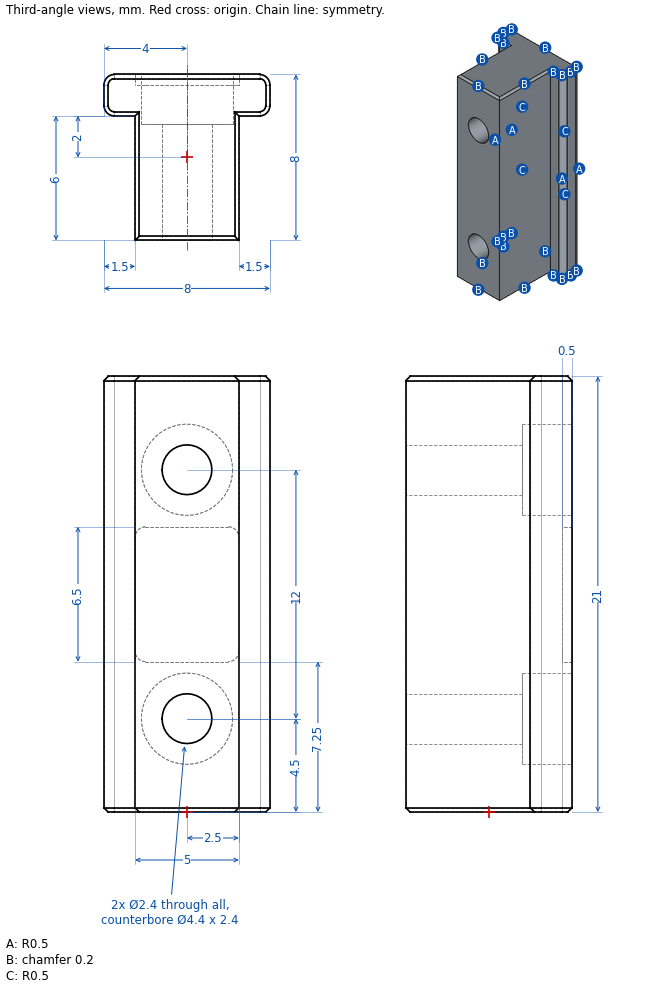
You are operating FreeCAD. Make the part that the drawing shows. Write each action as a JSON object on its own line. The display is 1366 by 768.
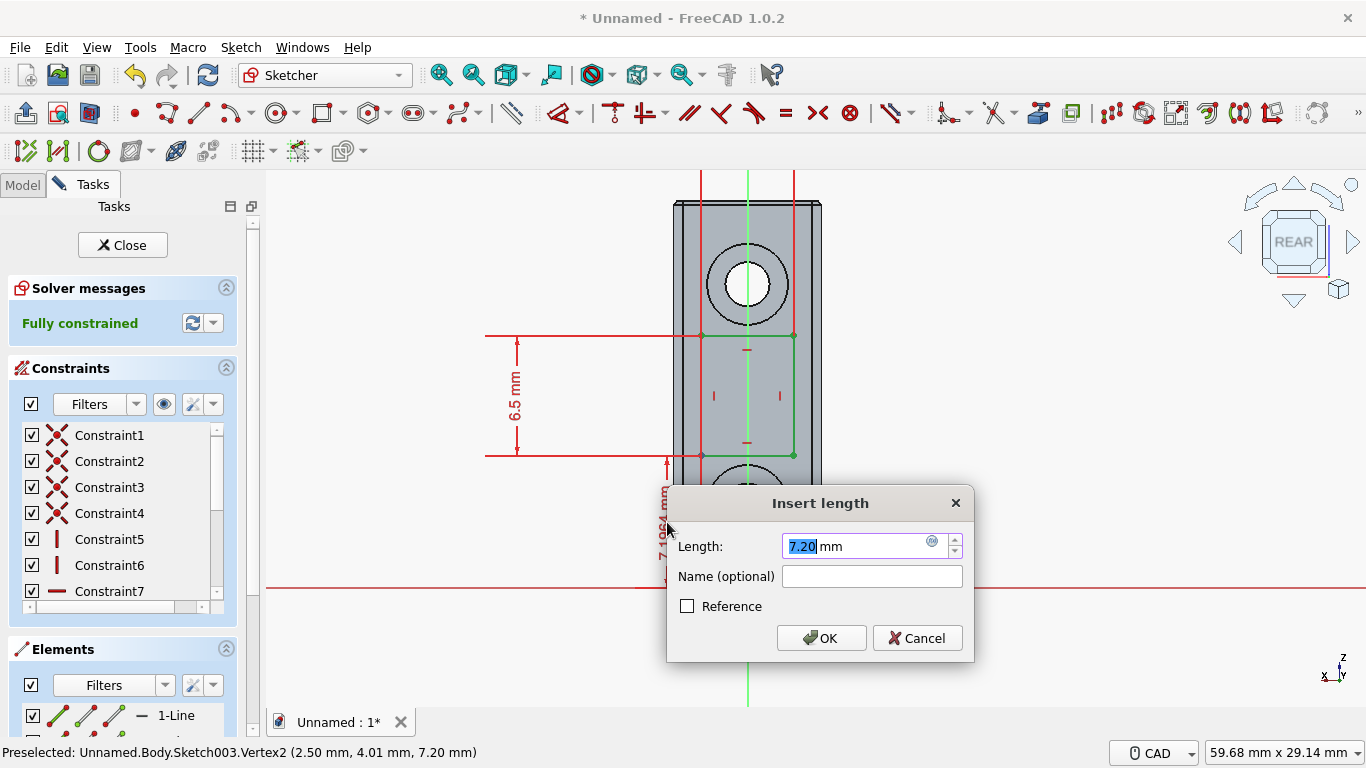
{"action": "type", "text": "7.25"}
{"action": "key", "text": "Return"}
{"action": "key", "text": "Escape"}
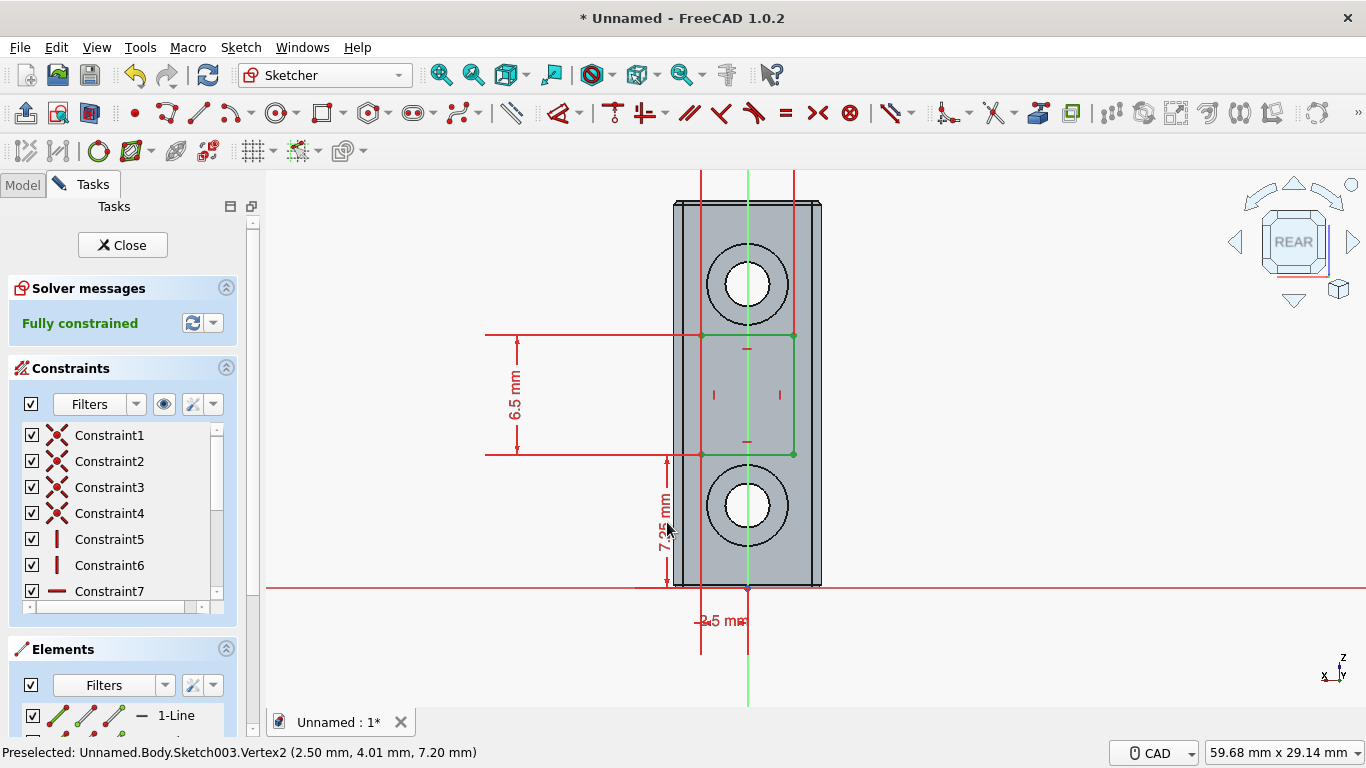
{"action": "left_click", "coordinate": [123, 245]}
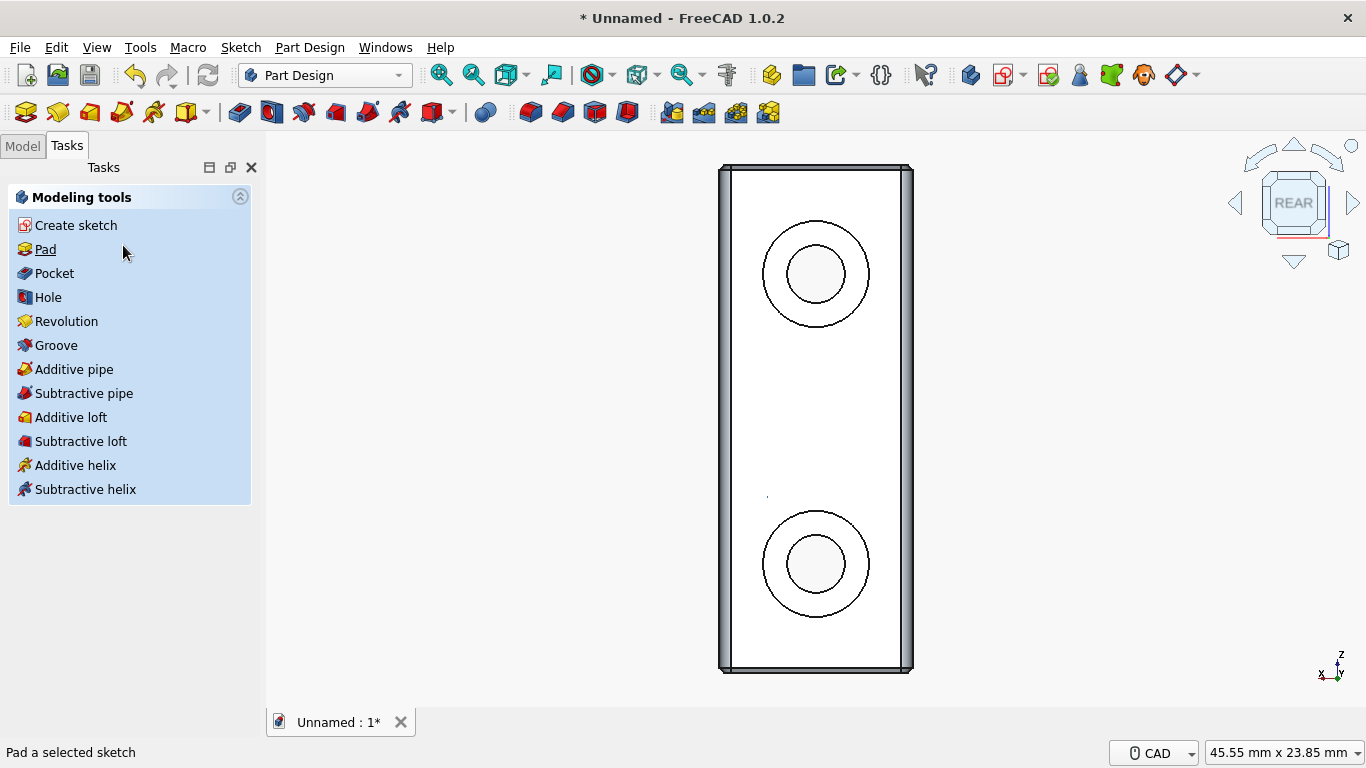
{"action": "left_click", "coordinate": [240, 112]}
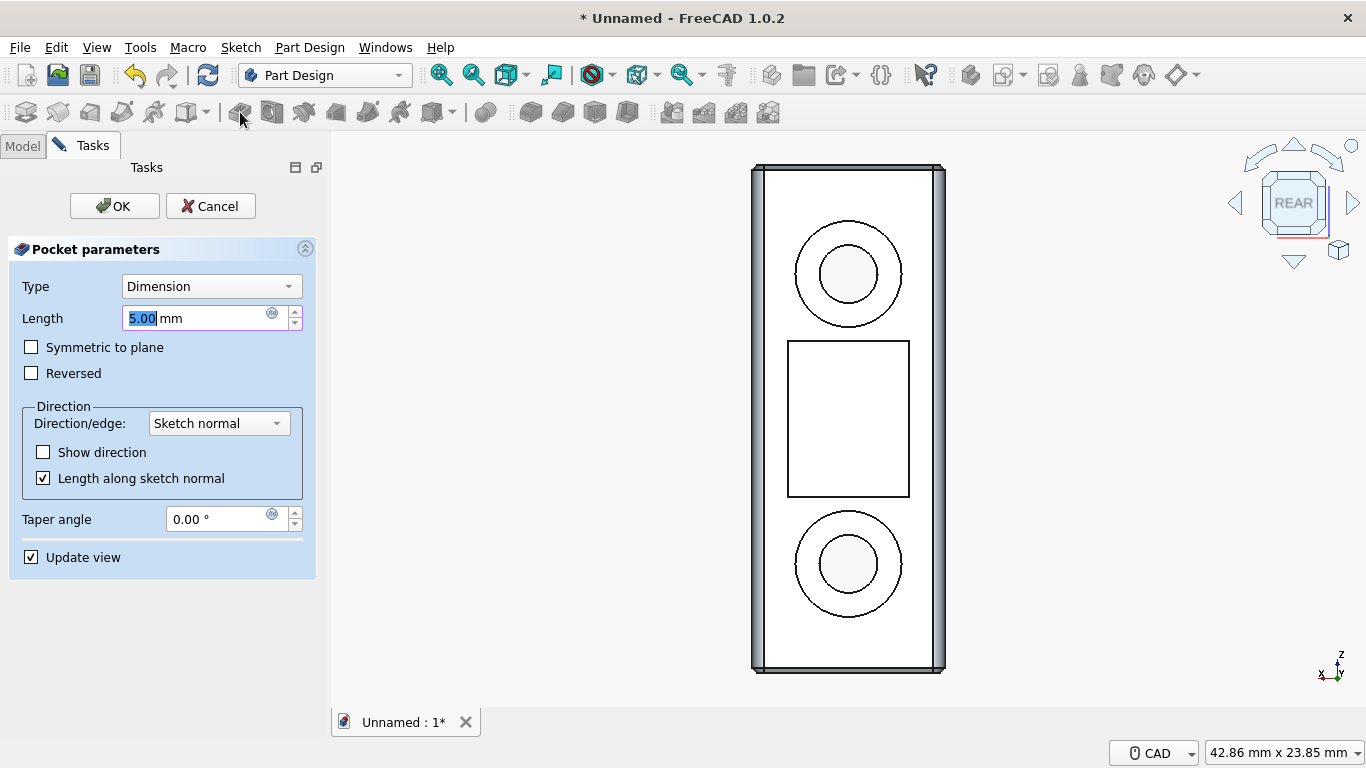
{"action": "type", "text": "0.5"}
{"action": "key", "text": "Tab"}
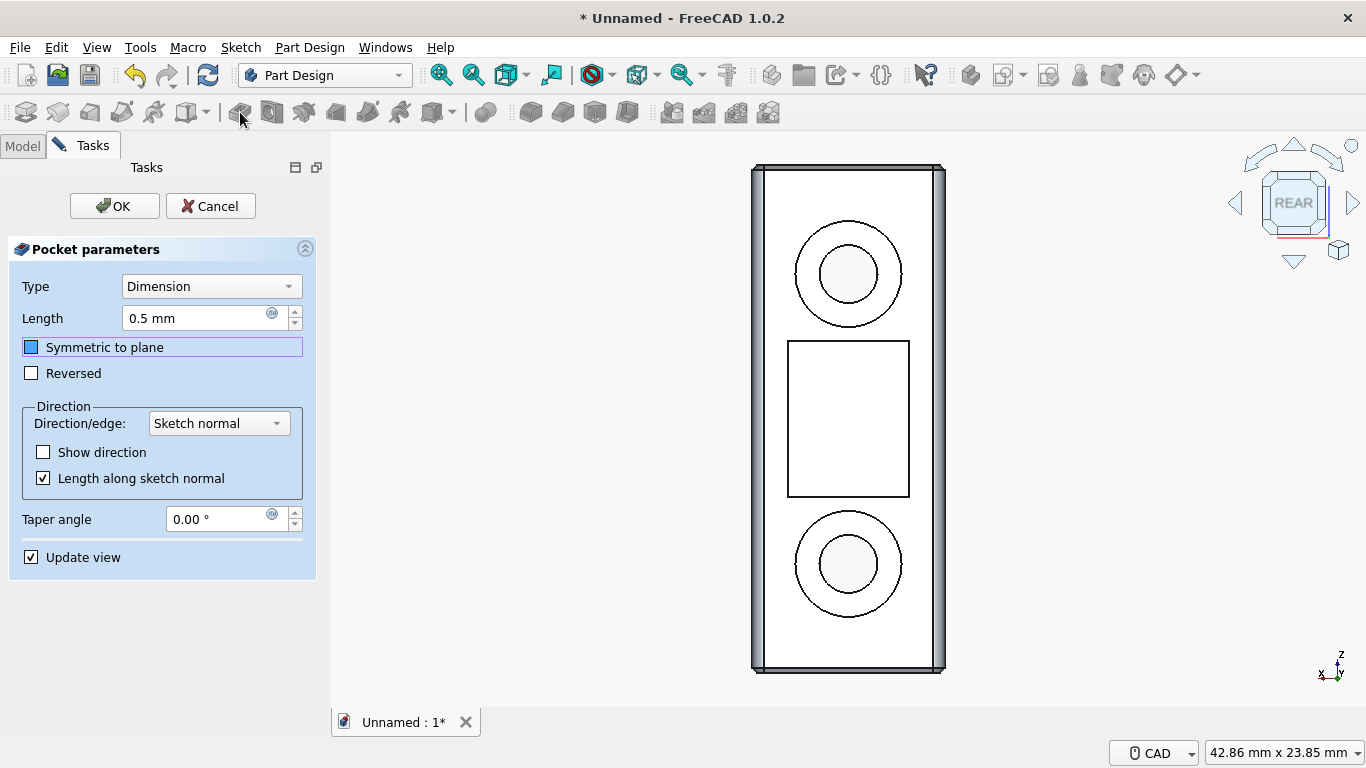
{"action": "left_click", "coordinate": [115, 206]}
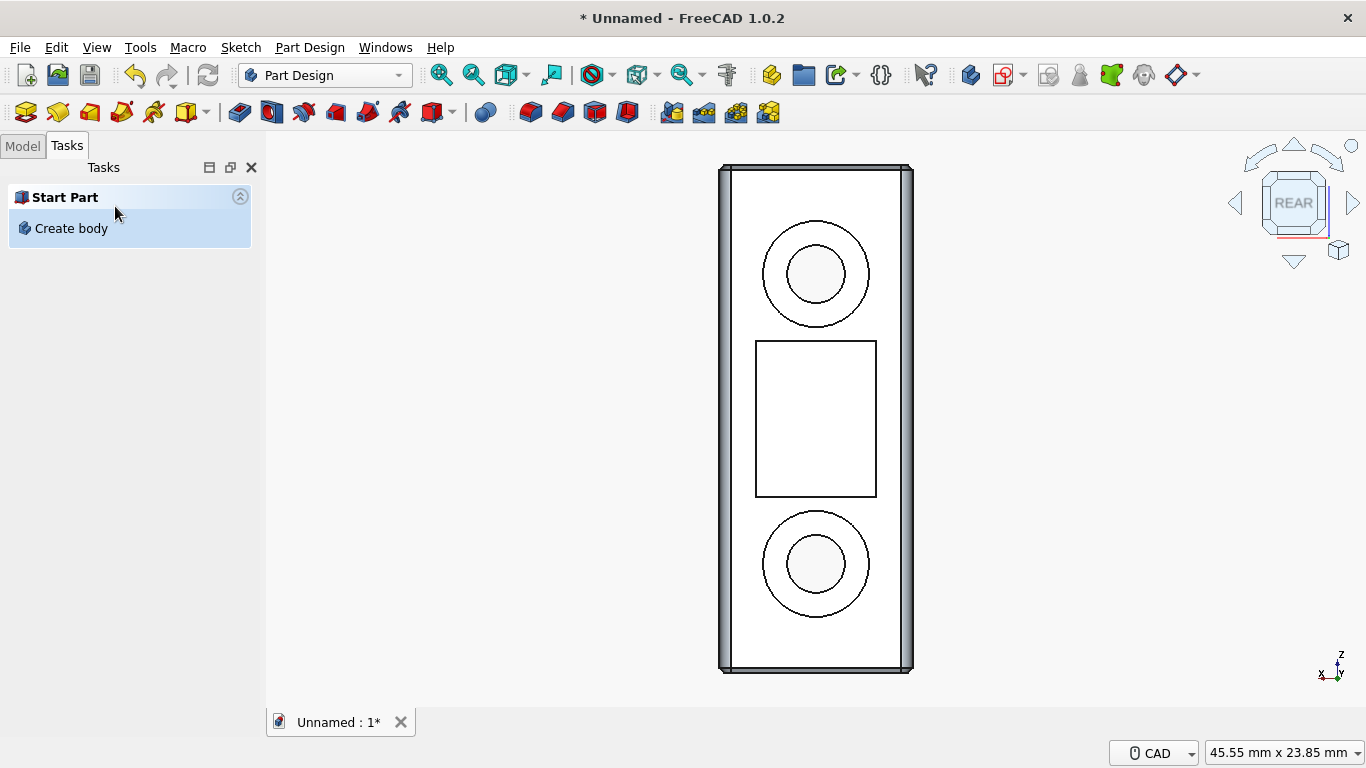
{"action": "scroll", "coordinate": [756, 496], "scroll_direction": "up", "scroll_amount": 6}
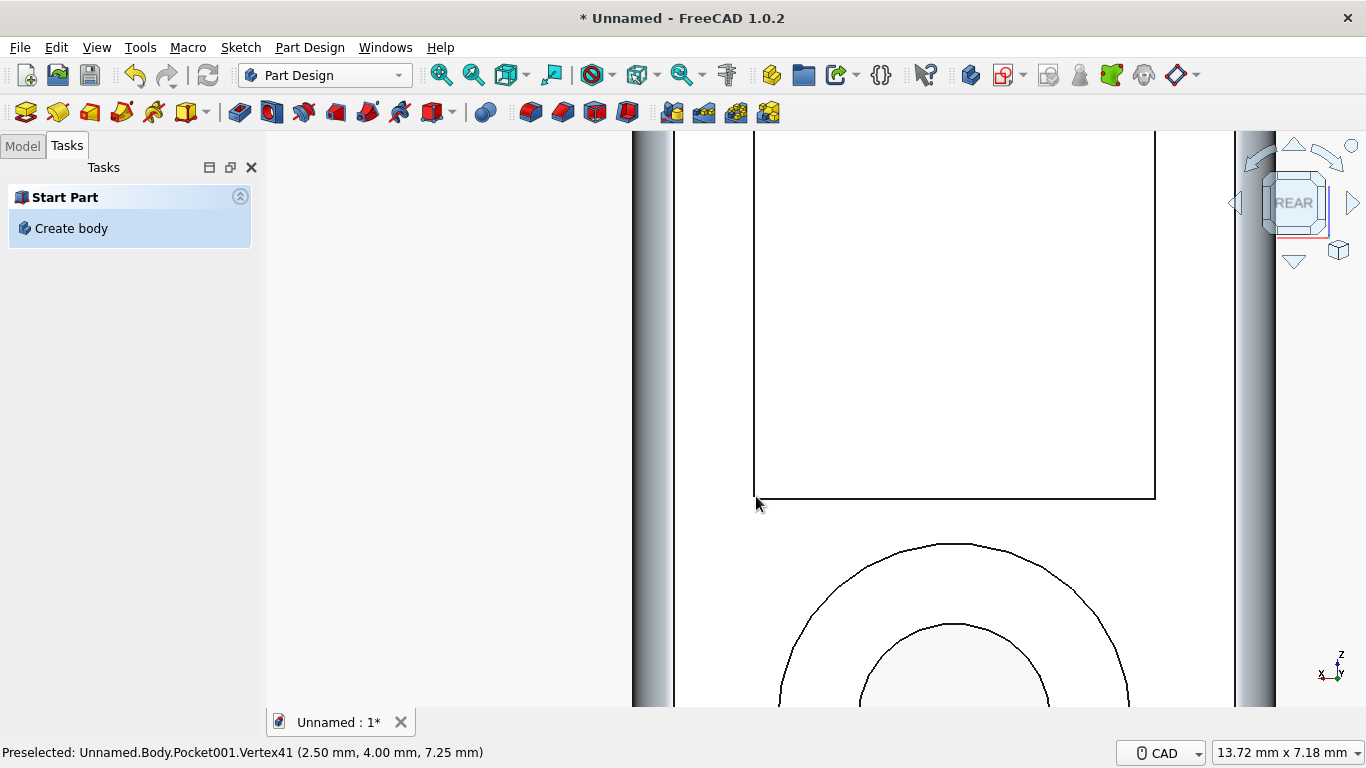
{"action": "left_click", "coordinate": [442, 76]}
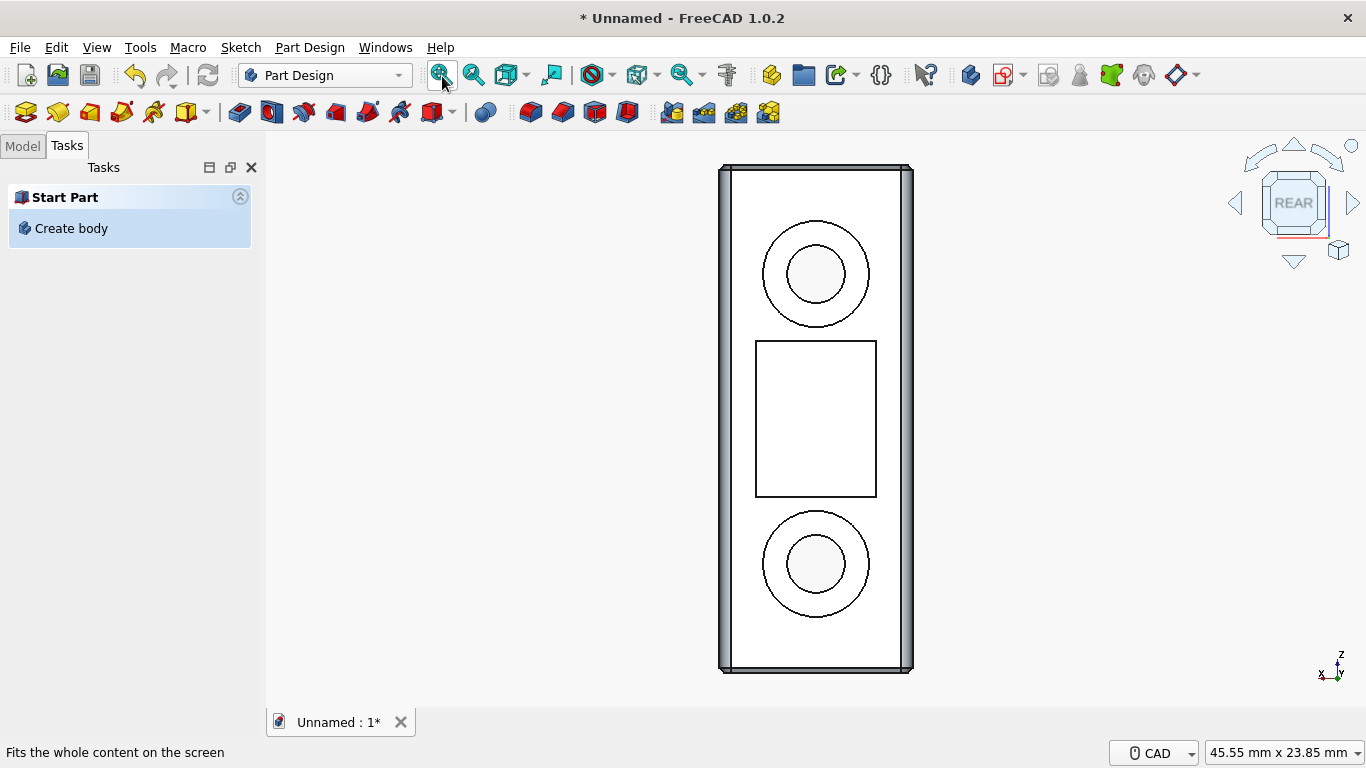
{"action": "key", "text": "0"}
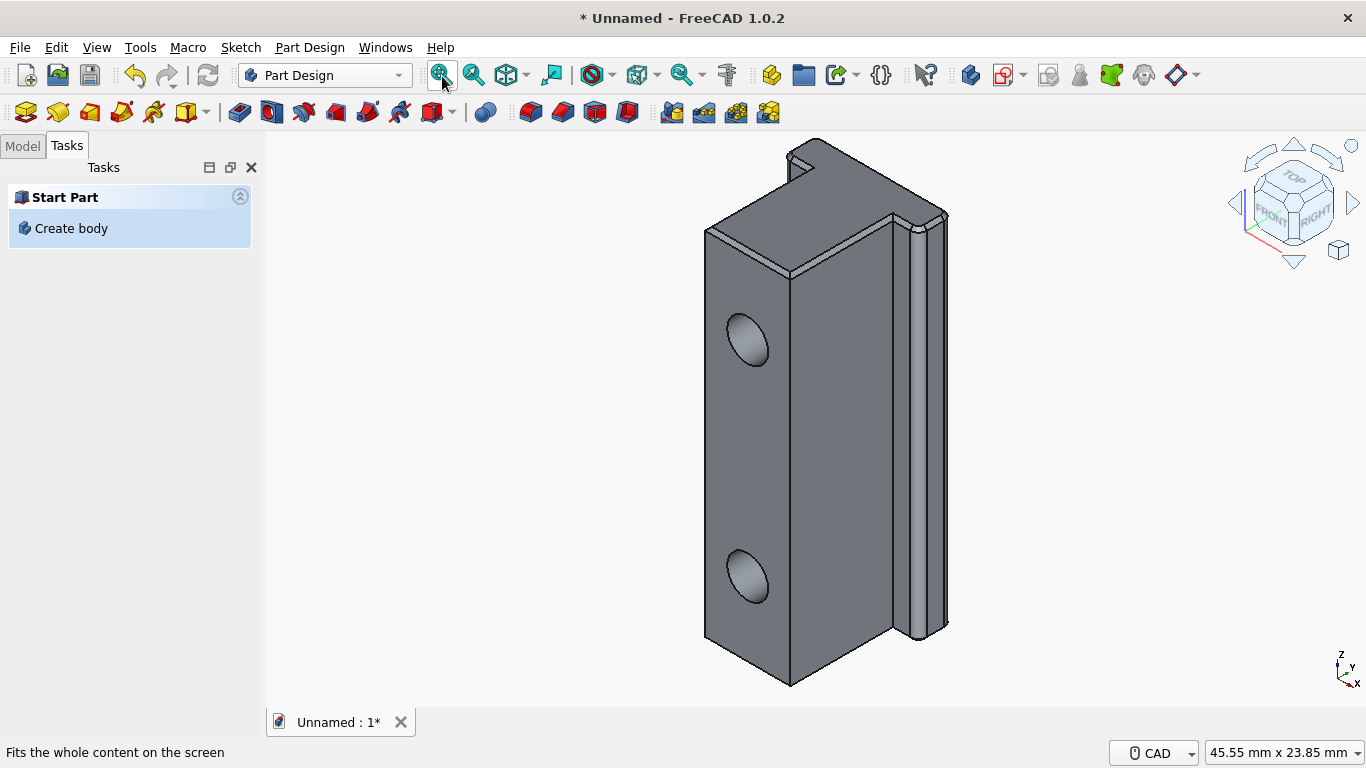
{"action": "scroll", "coordinate": [923, 470], "scroll_direction": "up", "scroll_amount": 6}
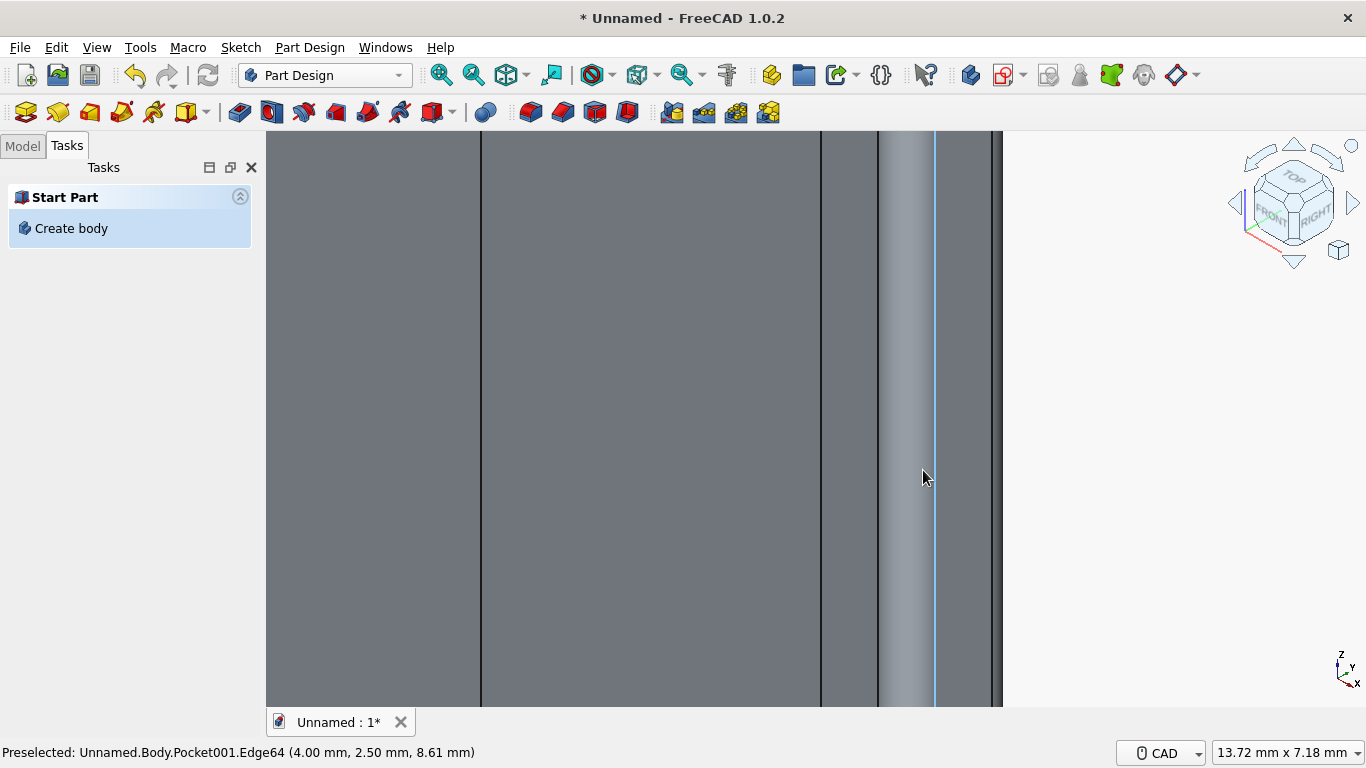
{"action": "left_click", "coordinate": [442, 76]}